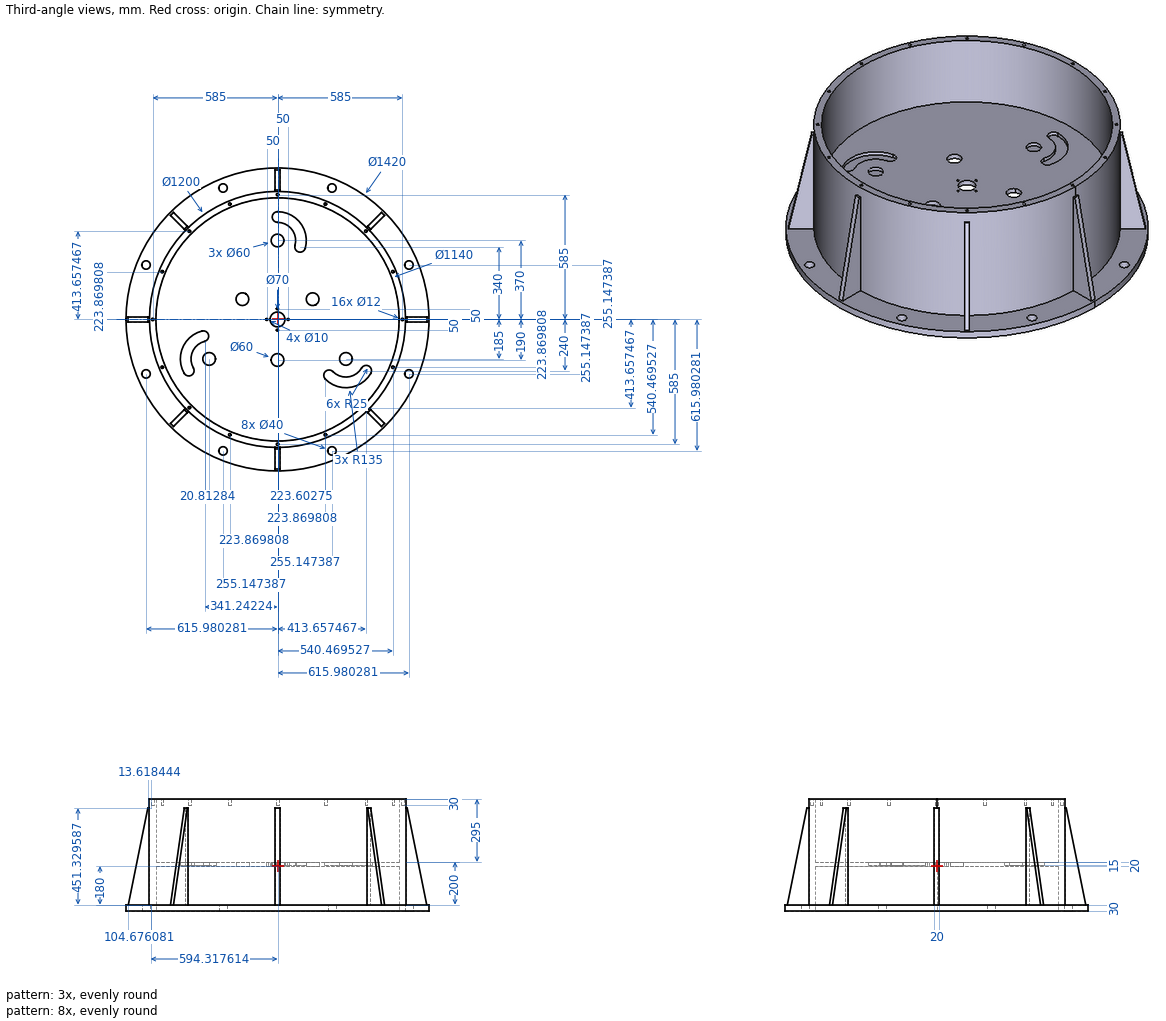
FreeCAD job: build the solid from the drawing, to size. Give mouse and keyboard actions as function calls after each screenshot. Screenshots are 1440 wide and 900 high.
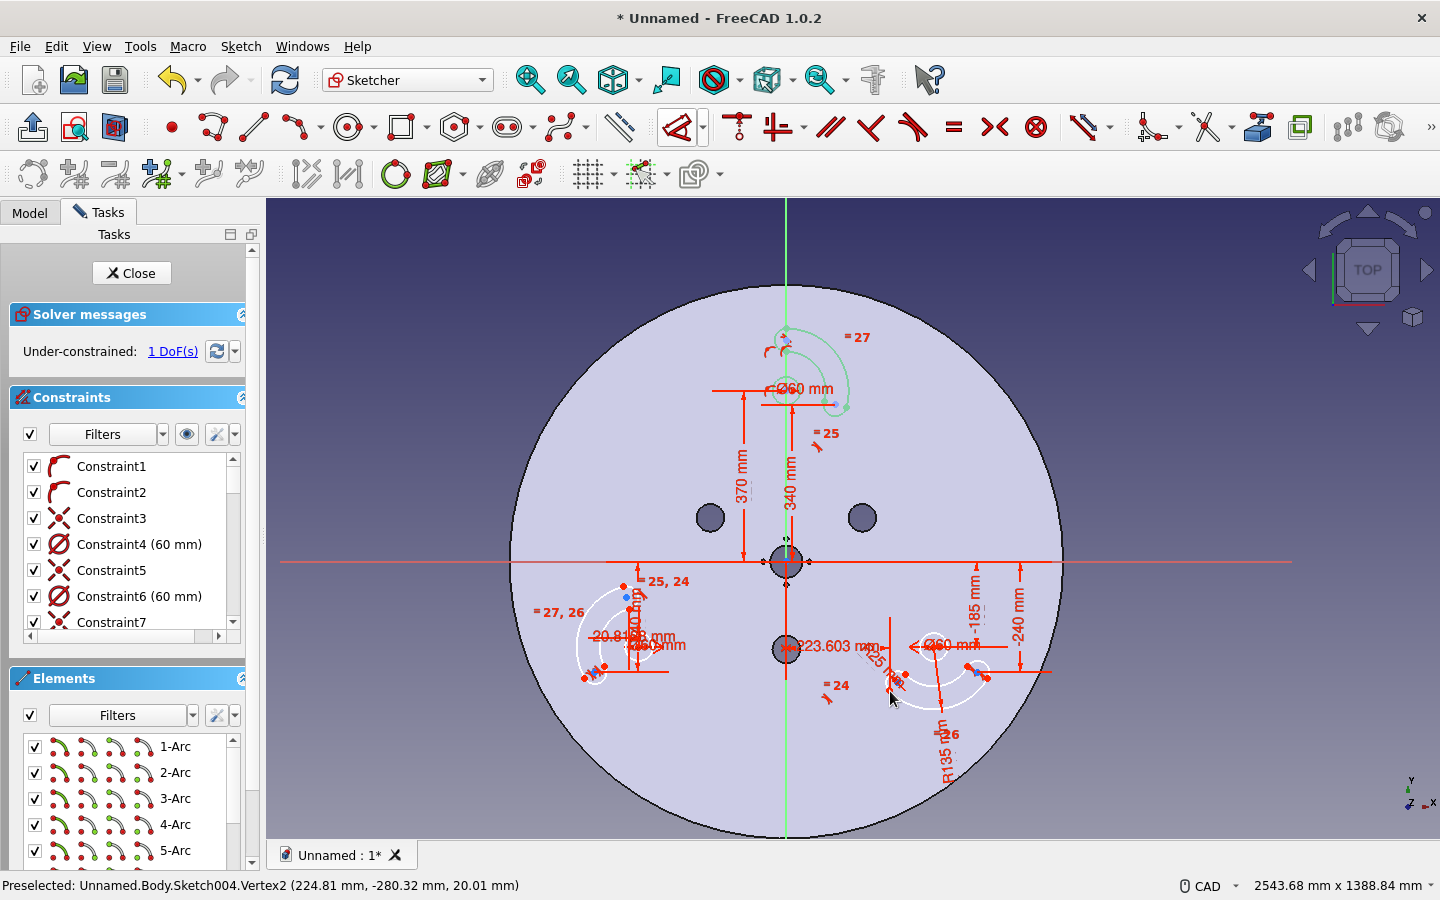
click(629, 609)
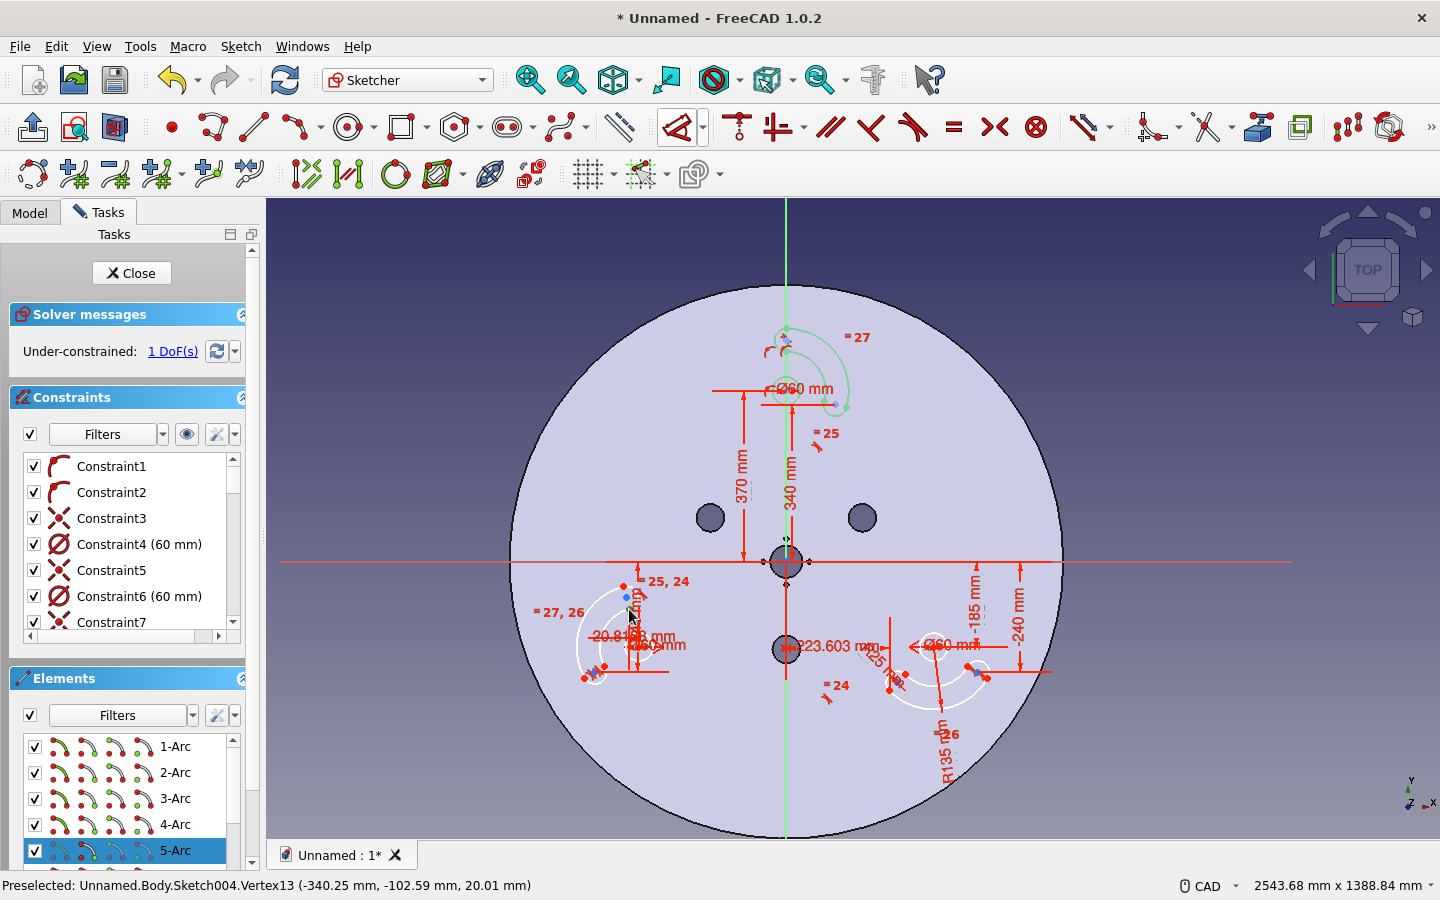
click(702, 128)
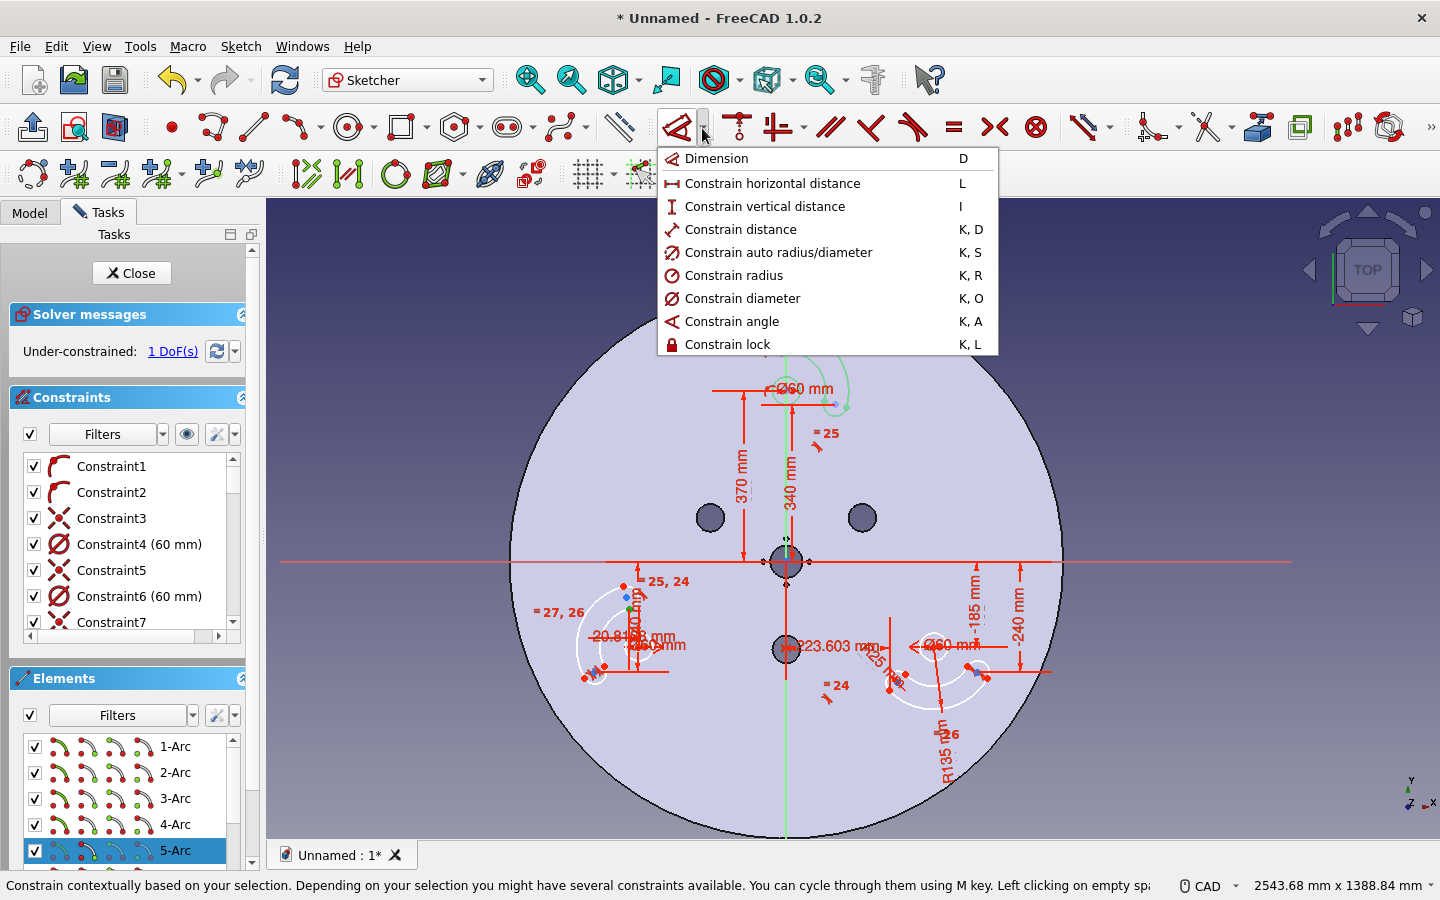
click(828, 184)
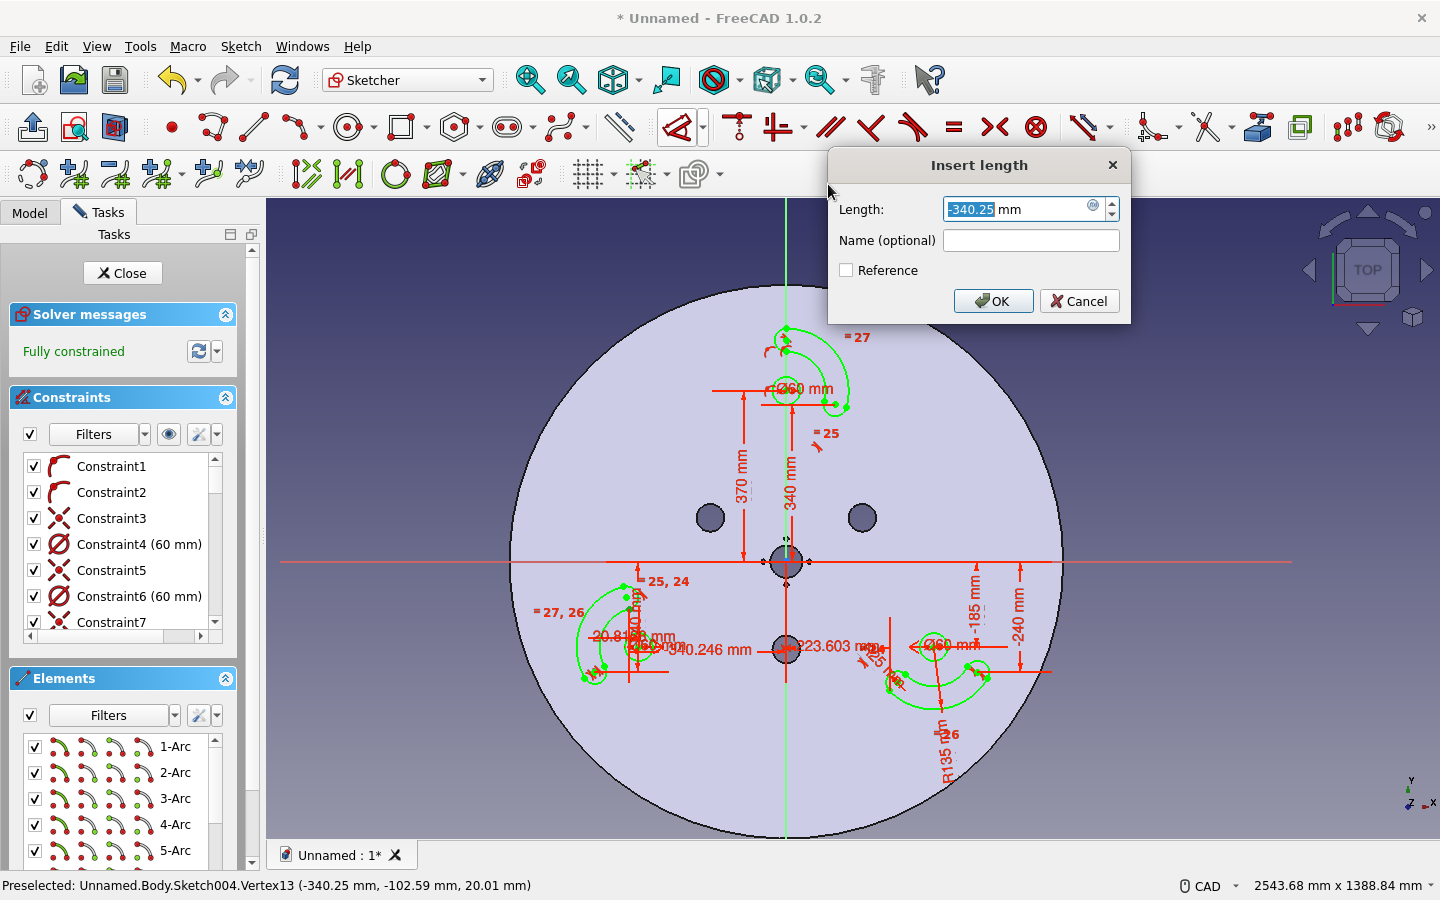
text(-341.24224)
key(Return)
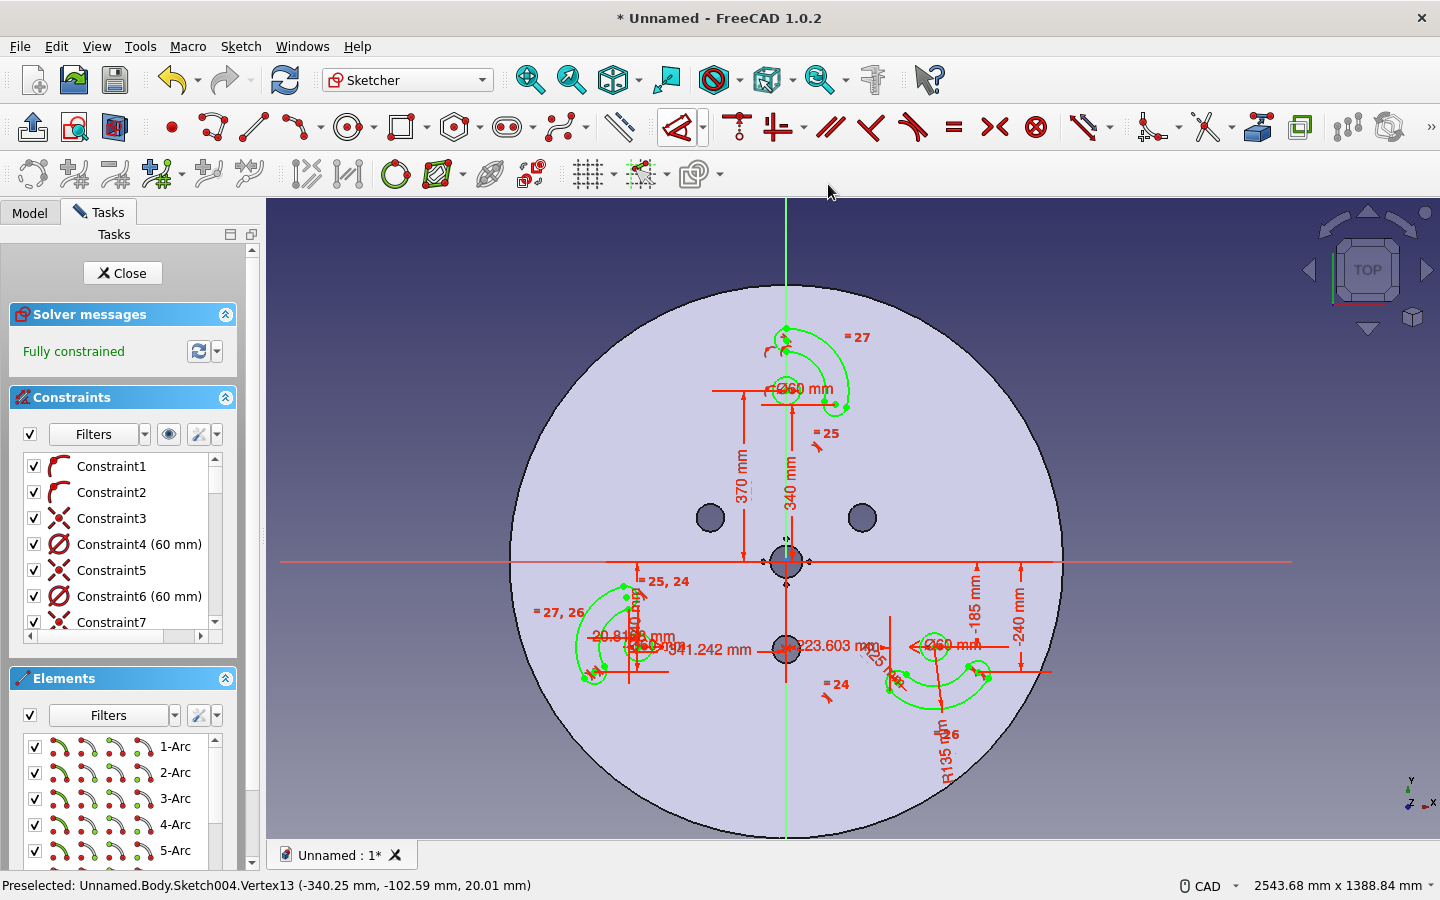
click(123, 273)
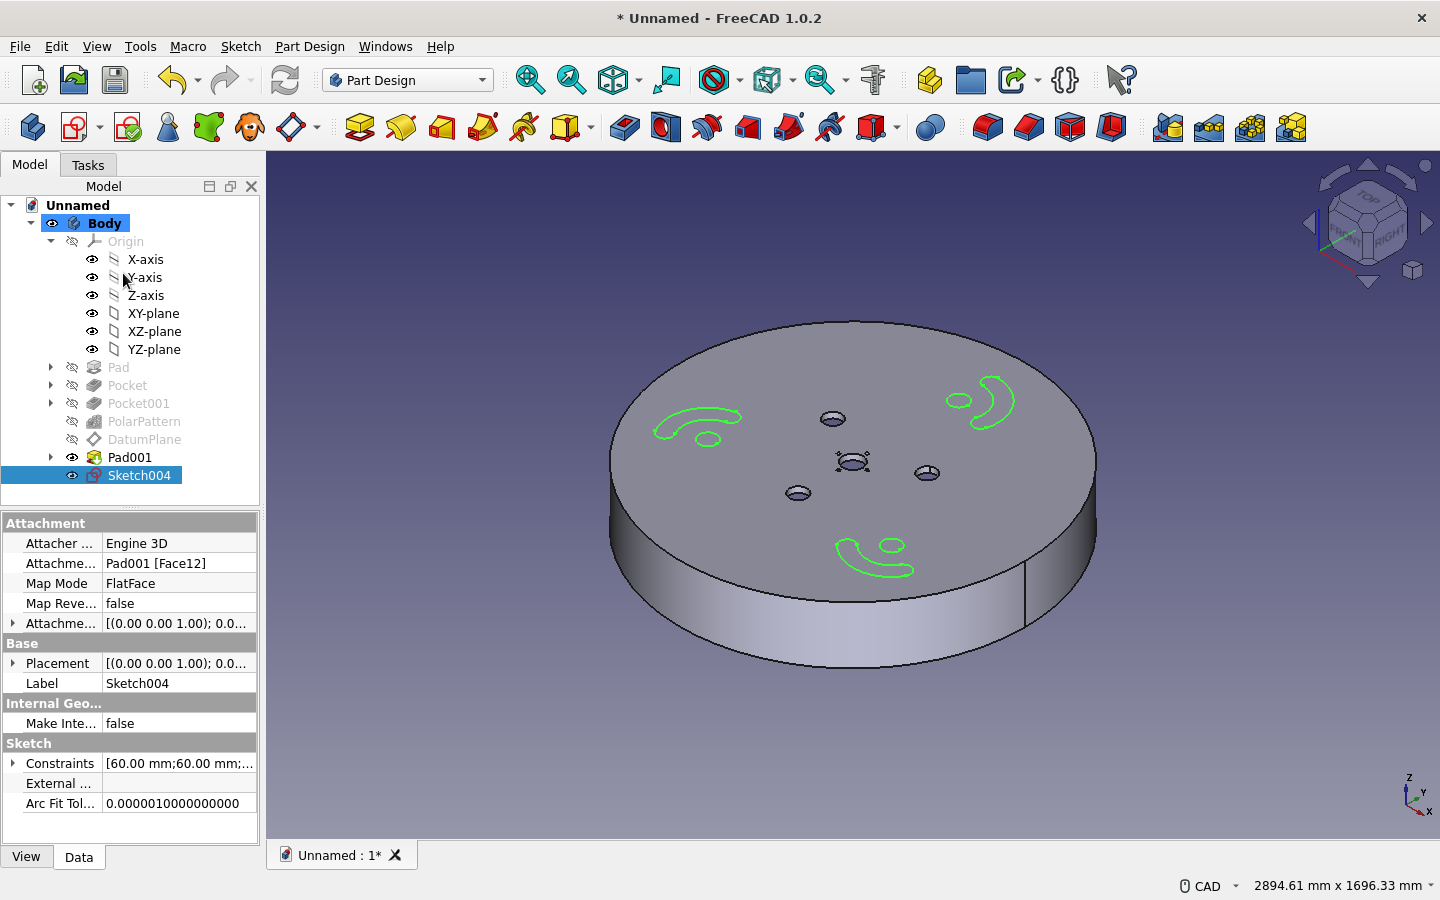
click(625, 128)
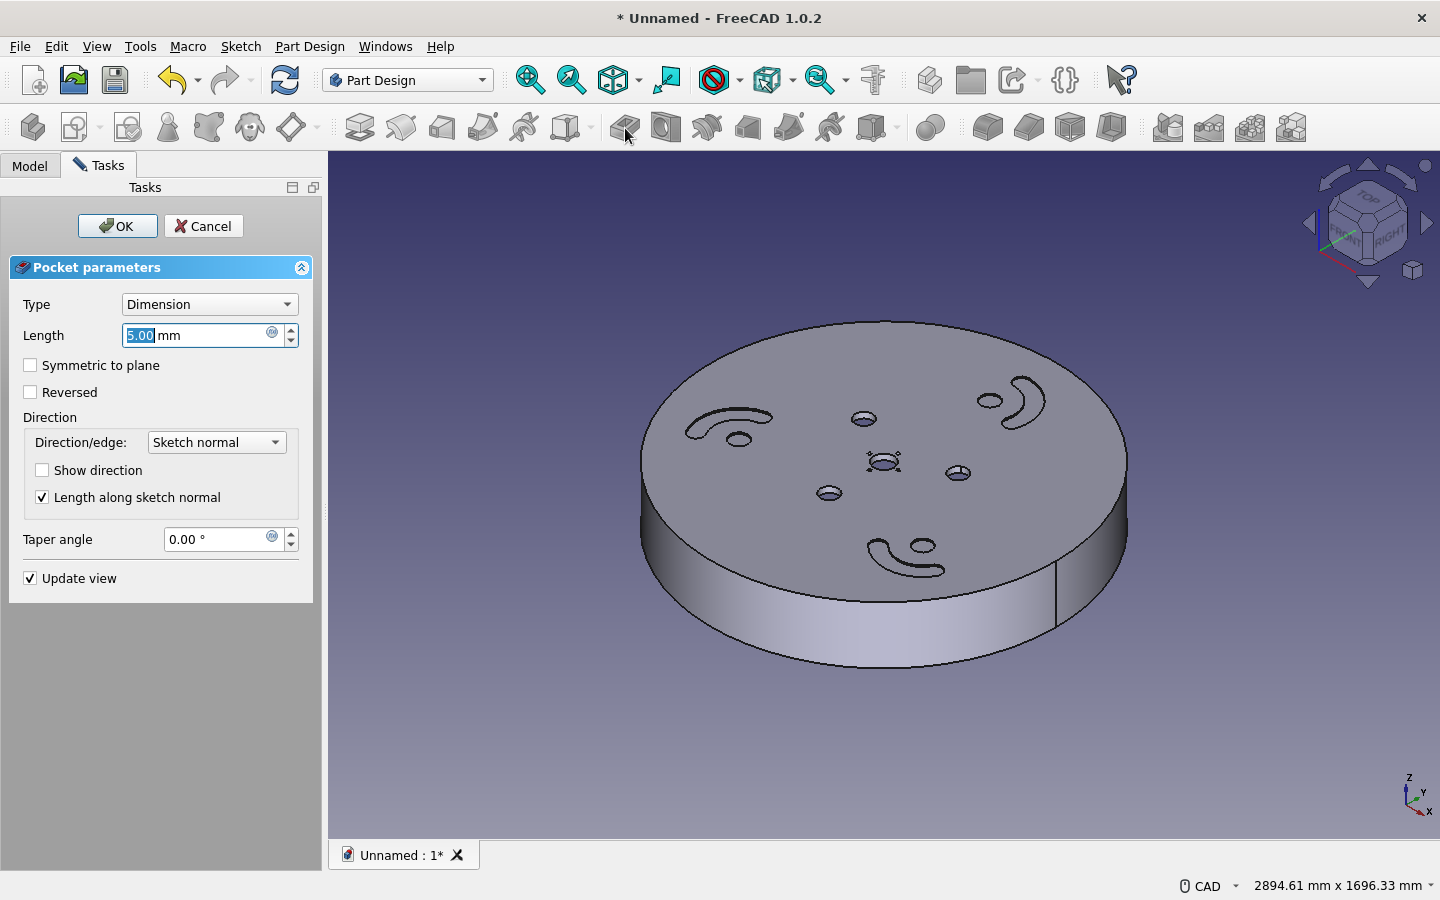
text(15)
key(Tab)